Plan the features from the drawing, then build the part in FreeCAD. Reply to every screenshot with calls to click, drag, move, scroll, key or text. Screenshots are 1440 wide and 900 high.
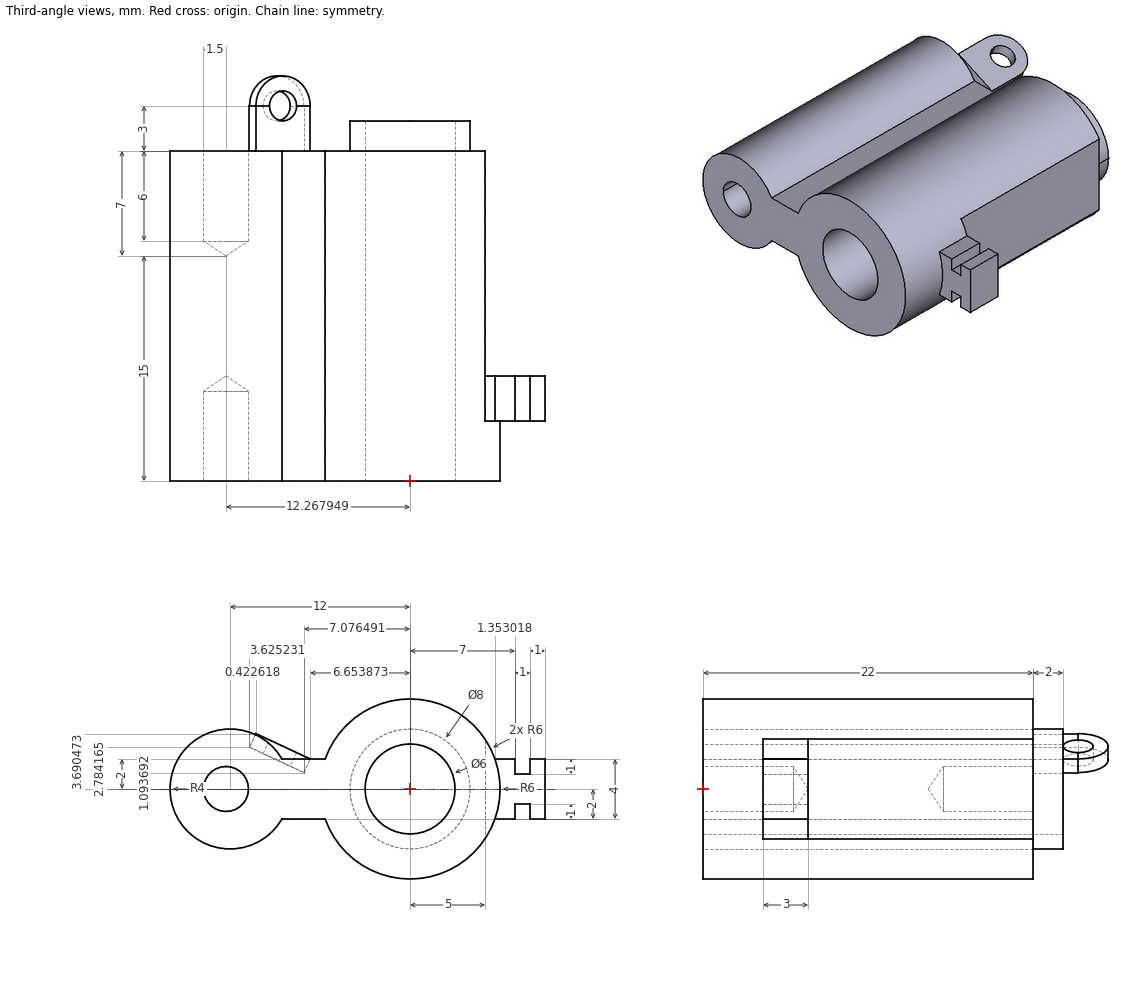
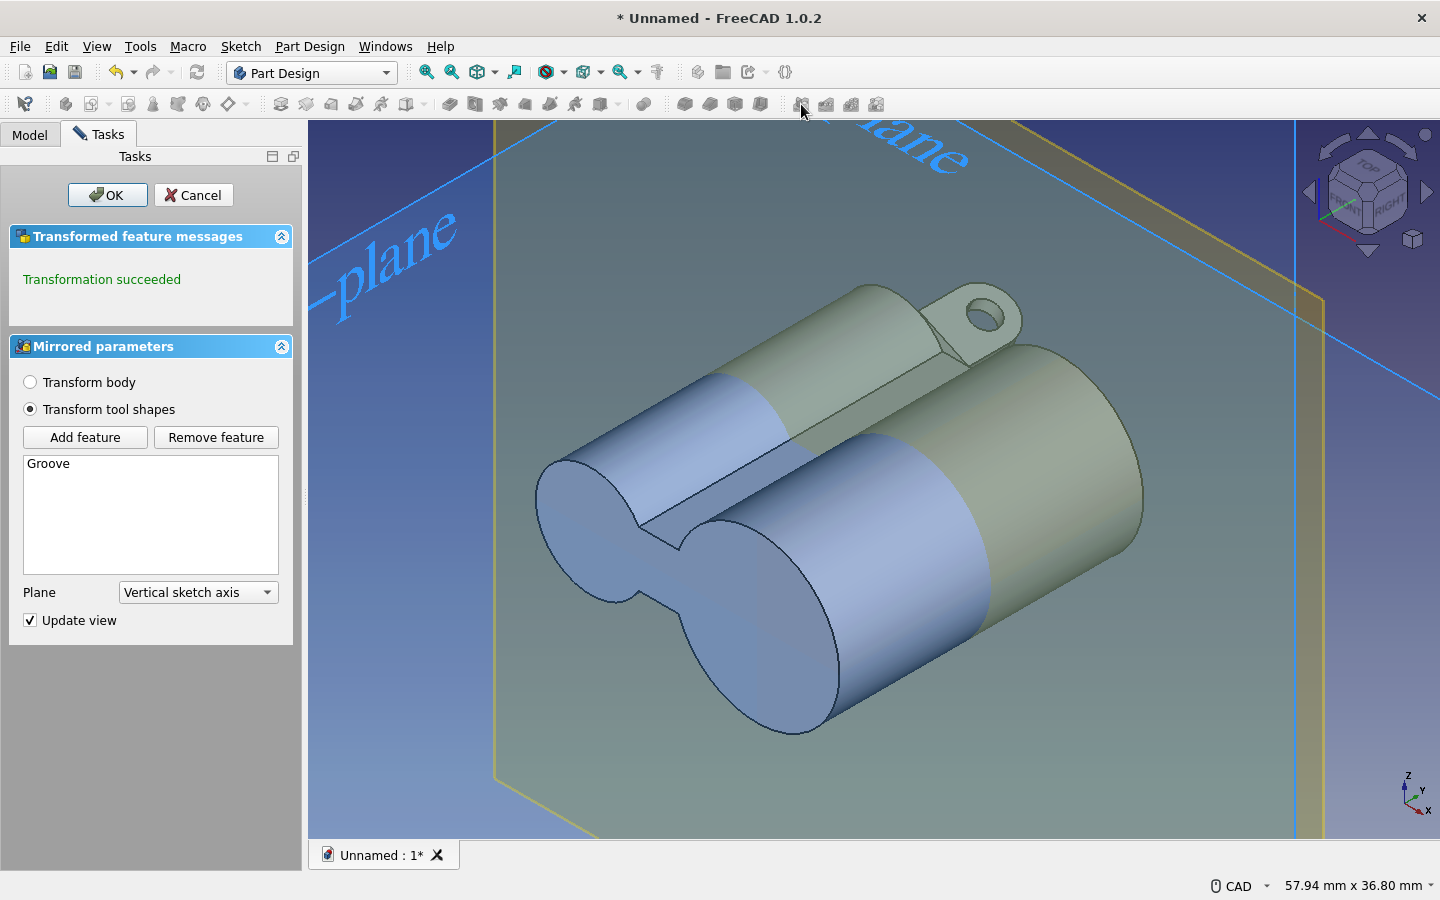
click(199, 592)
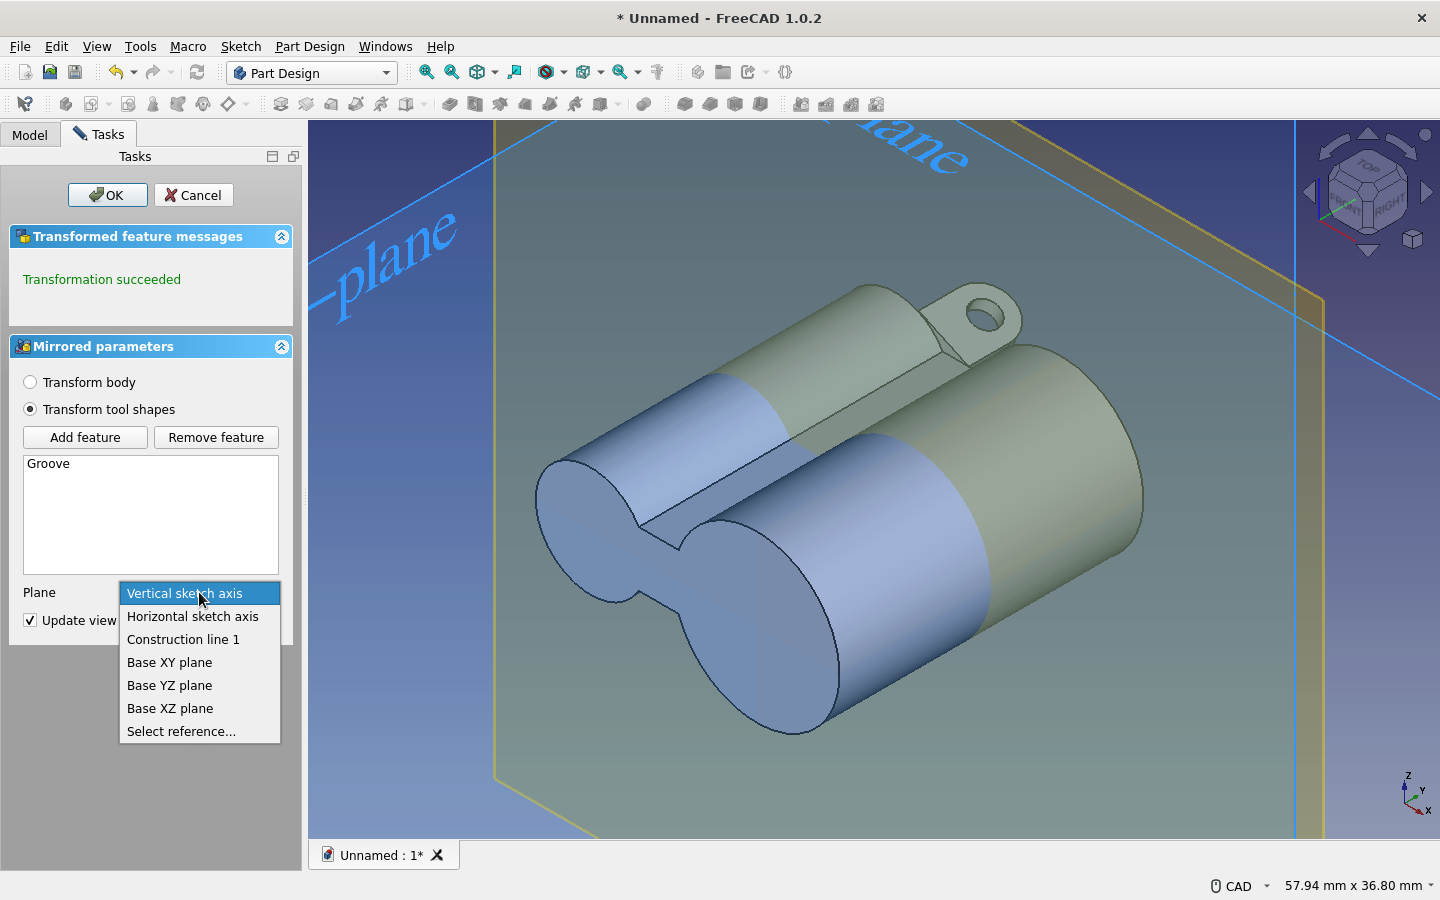
click(198, 732)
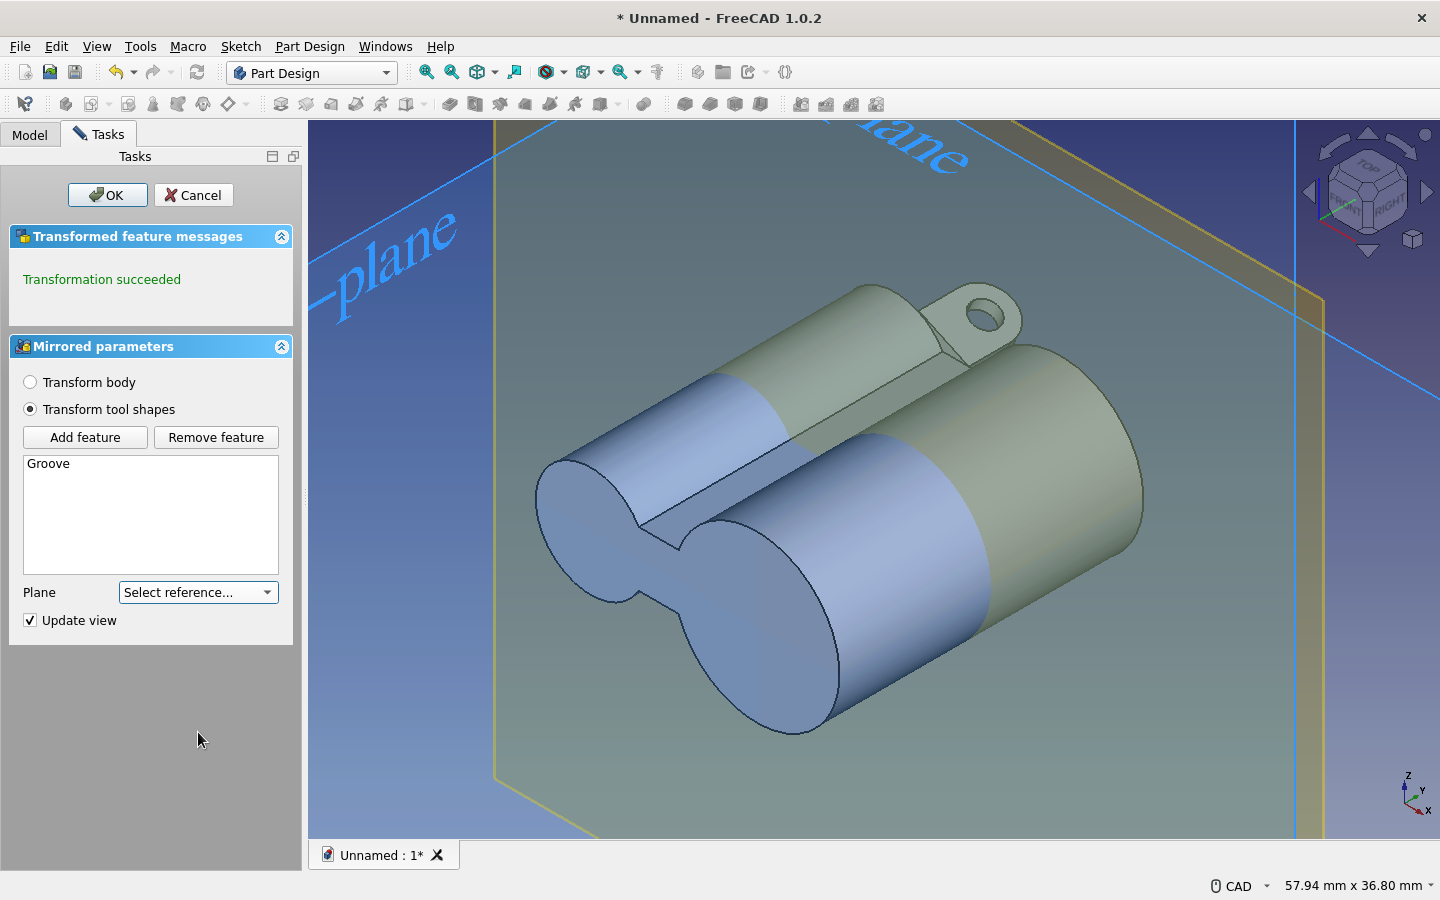
click(30, 134)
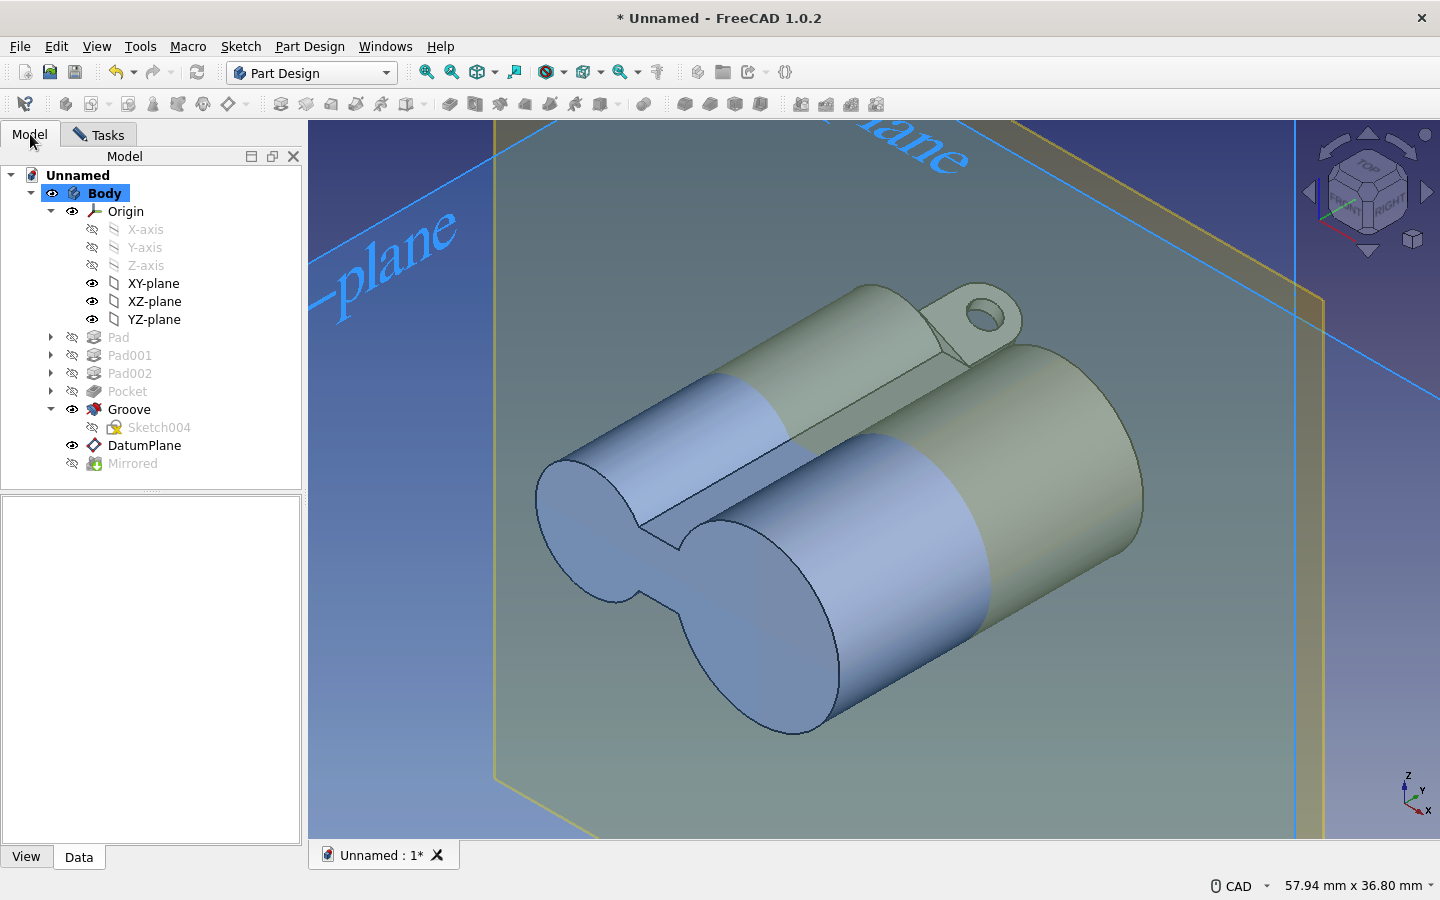
click(117, 445)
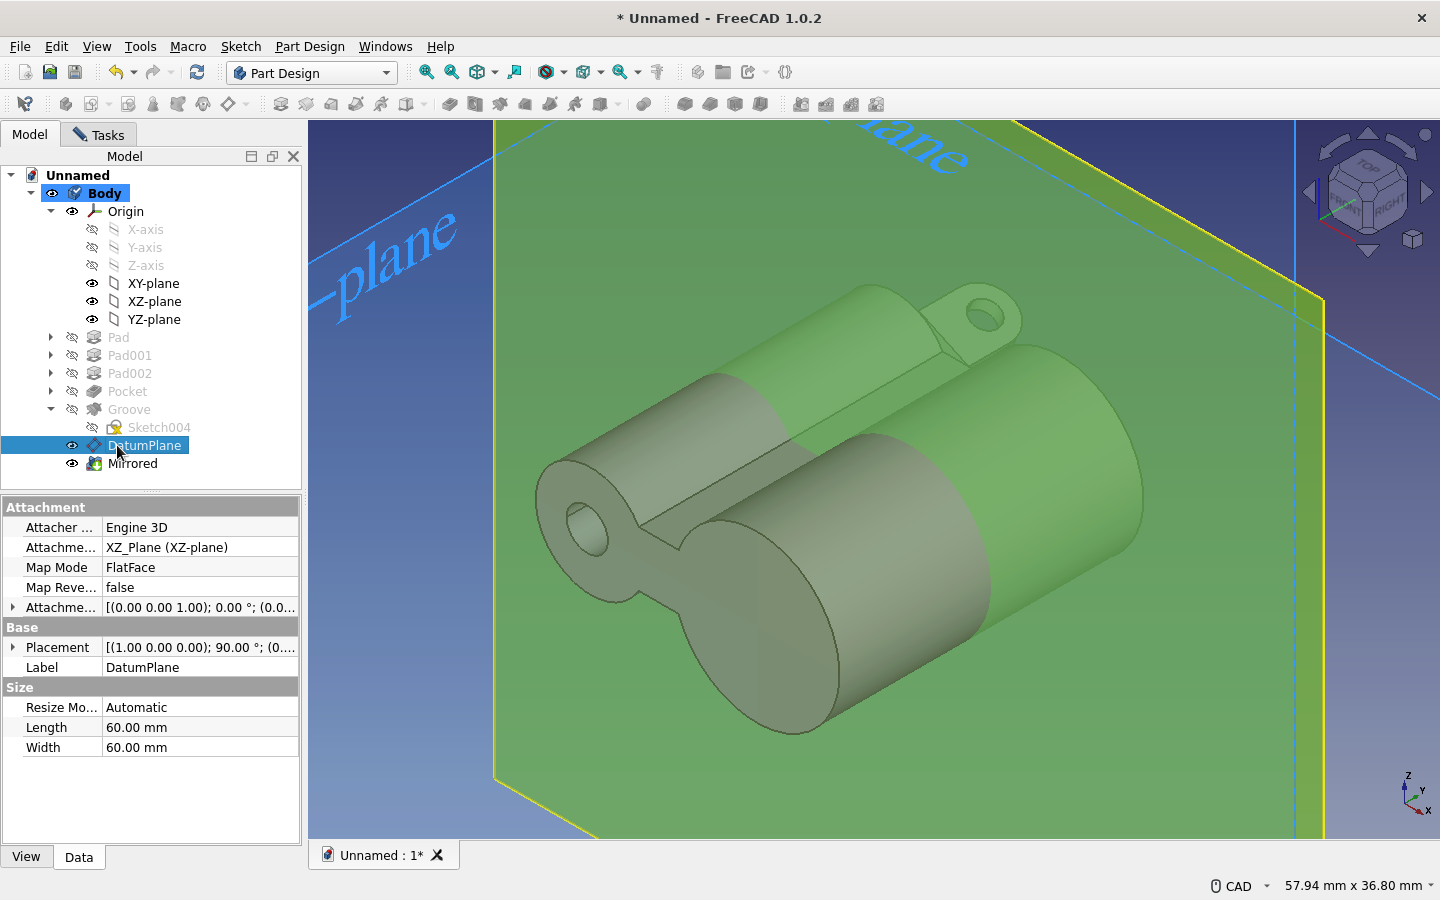
click(98, 134)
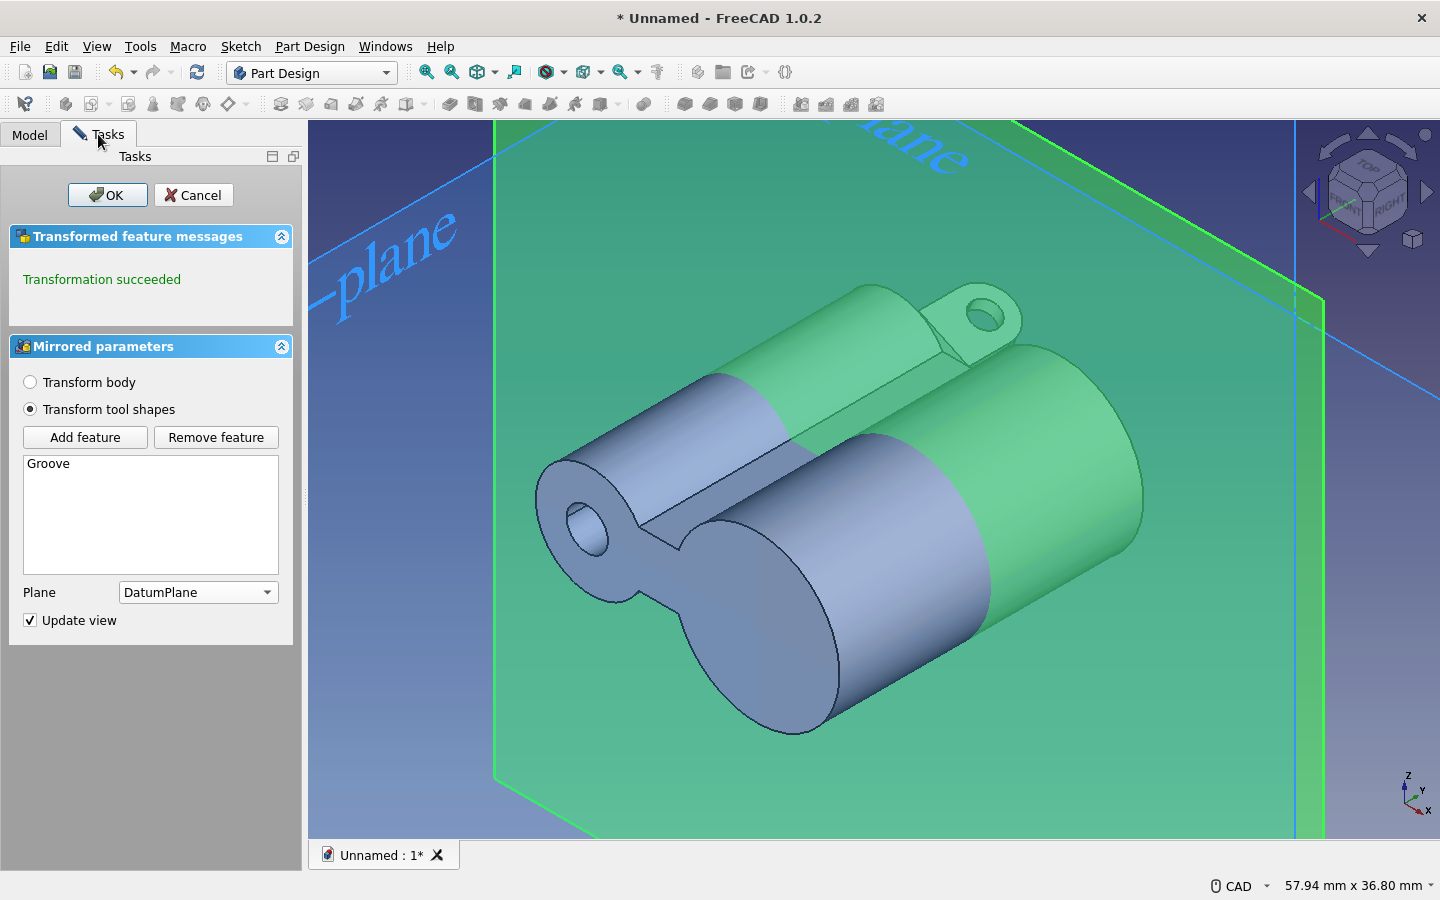
click(108, 195)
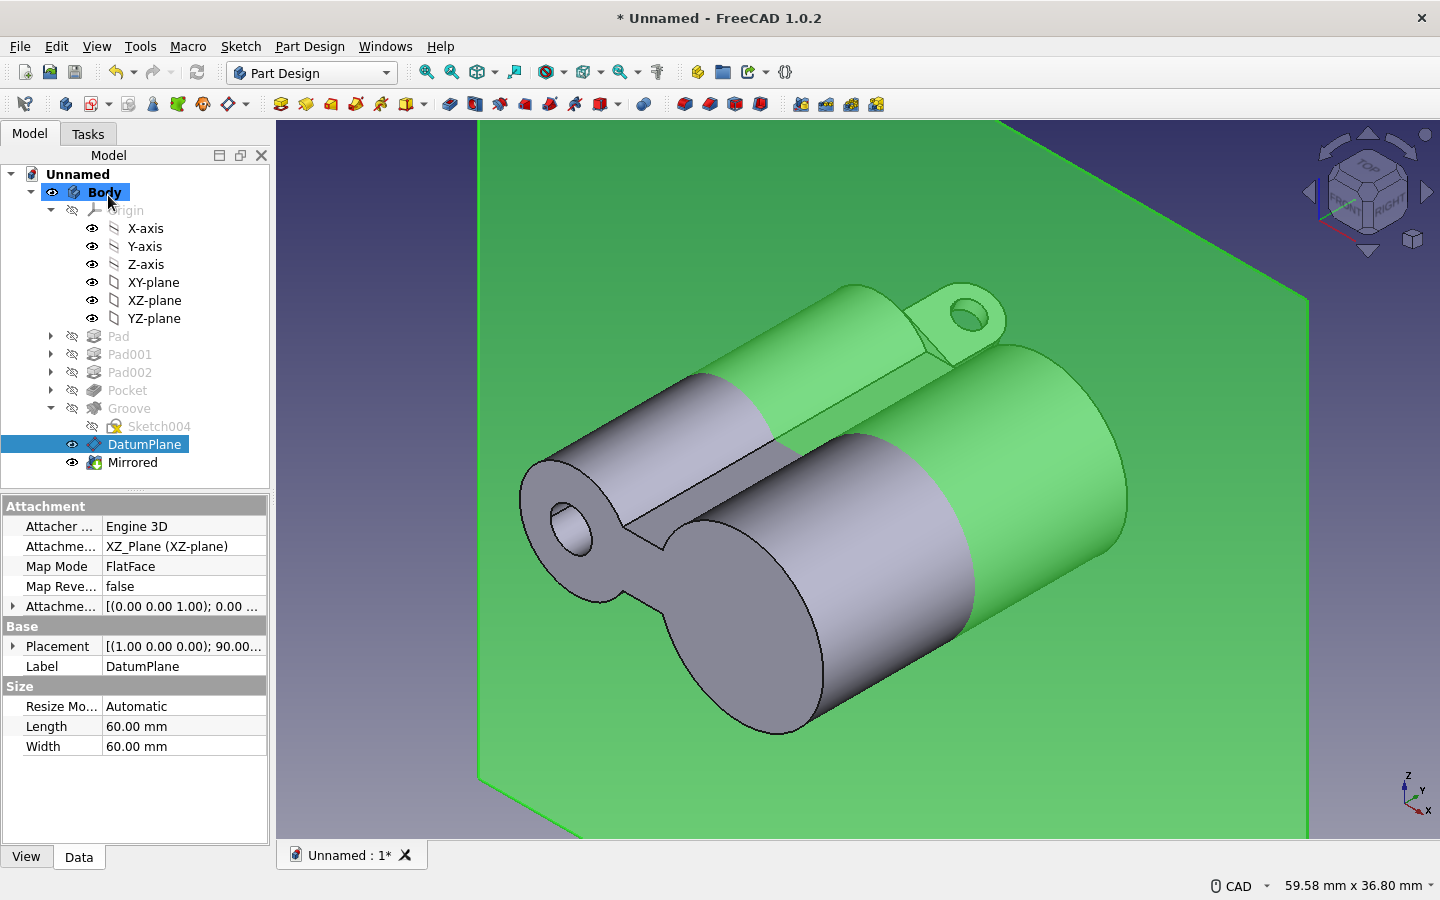
click(117, 444)
key(space)